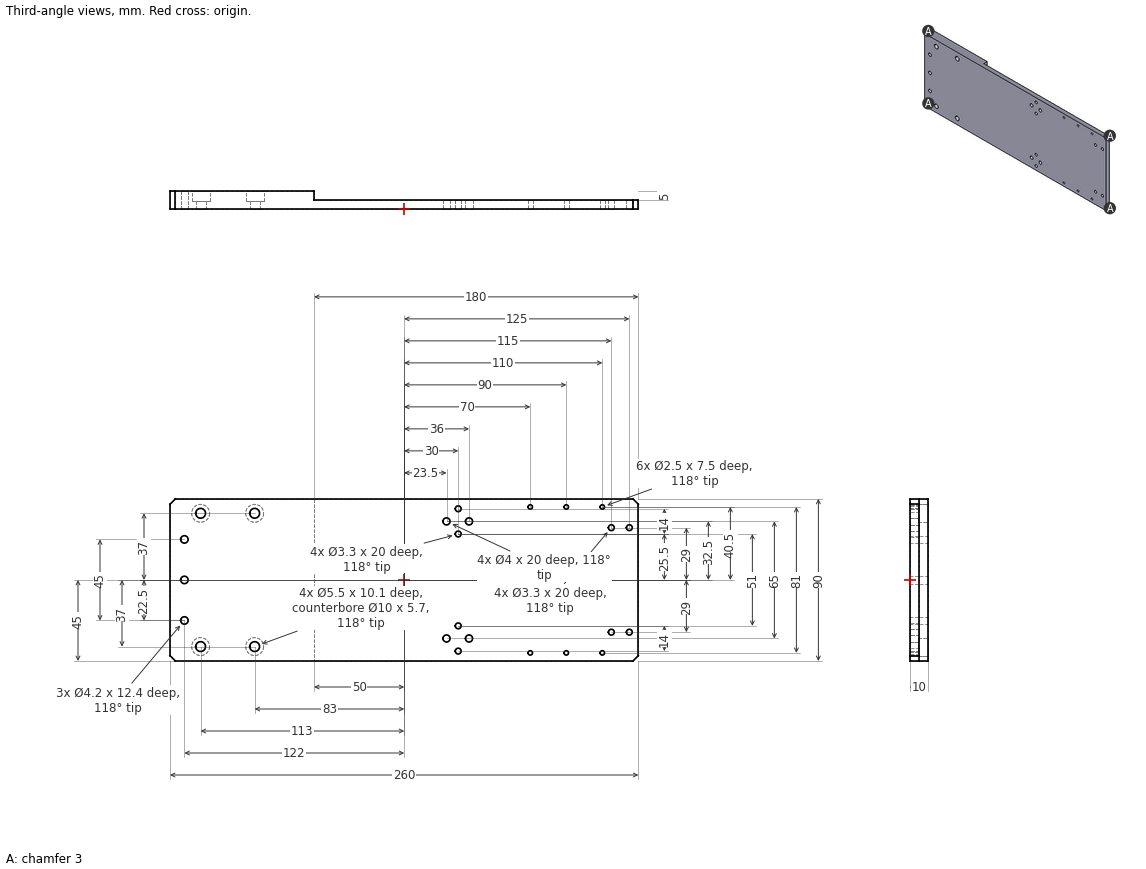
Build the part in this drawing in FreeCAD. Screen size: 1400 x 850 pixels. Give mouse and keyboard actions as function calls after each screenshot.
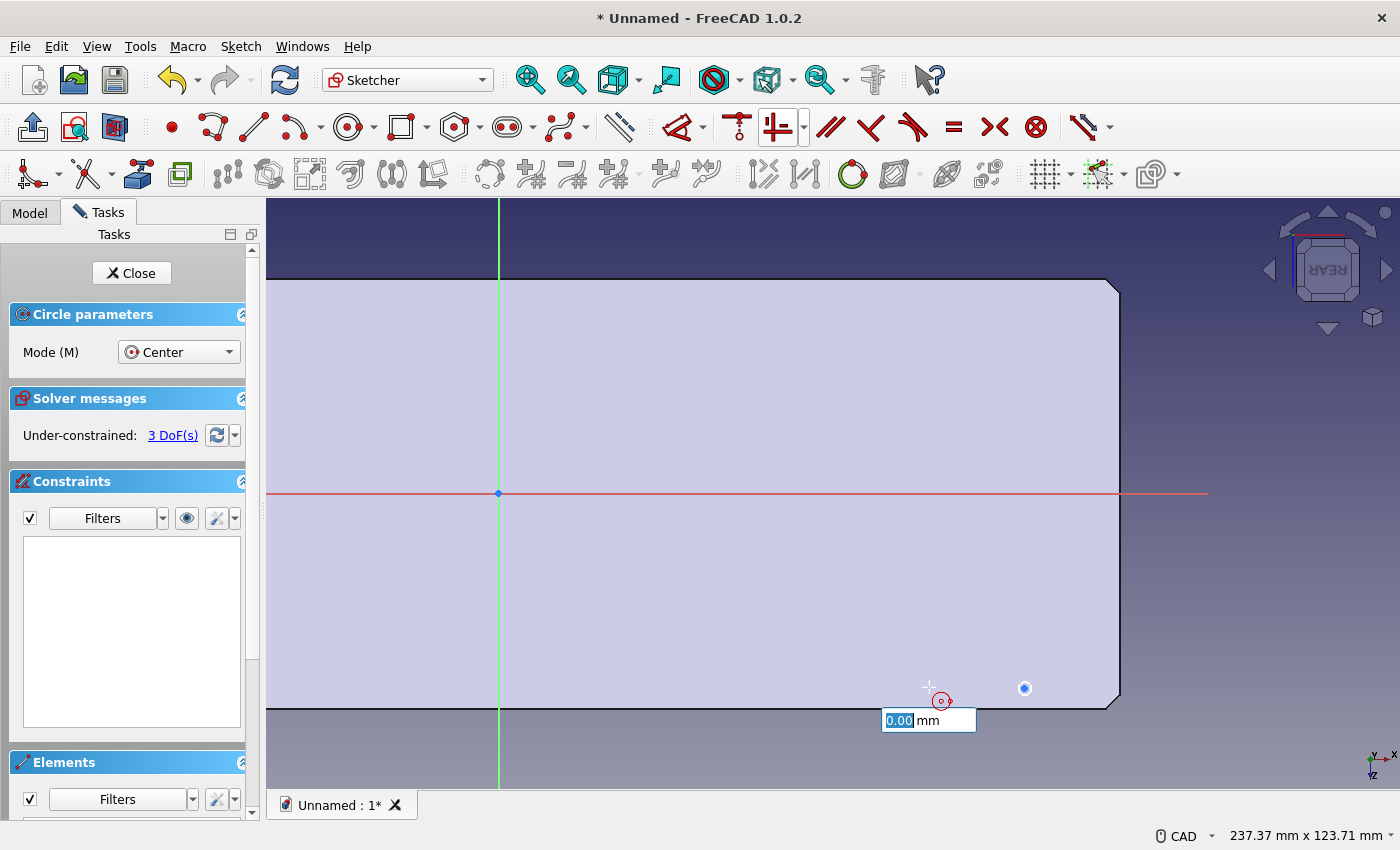
scroll(933, 683, up, 5)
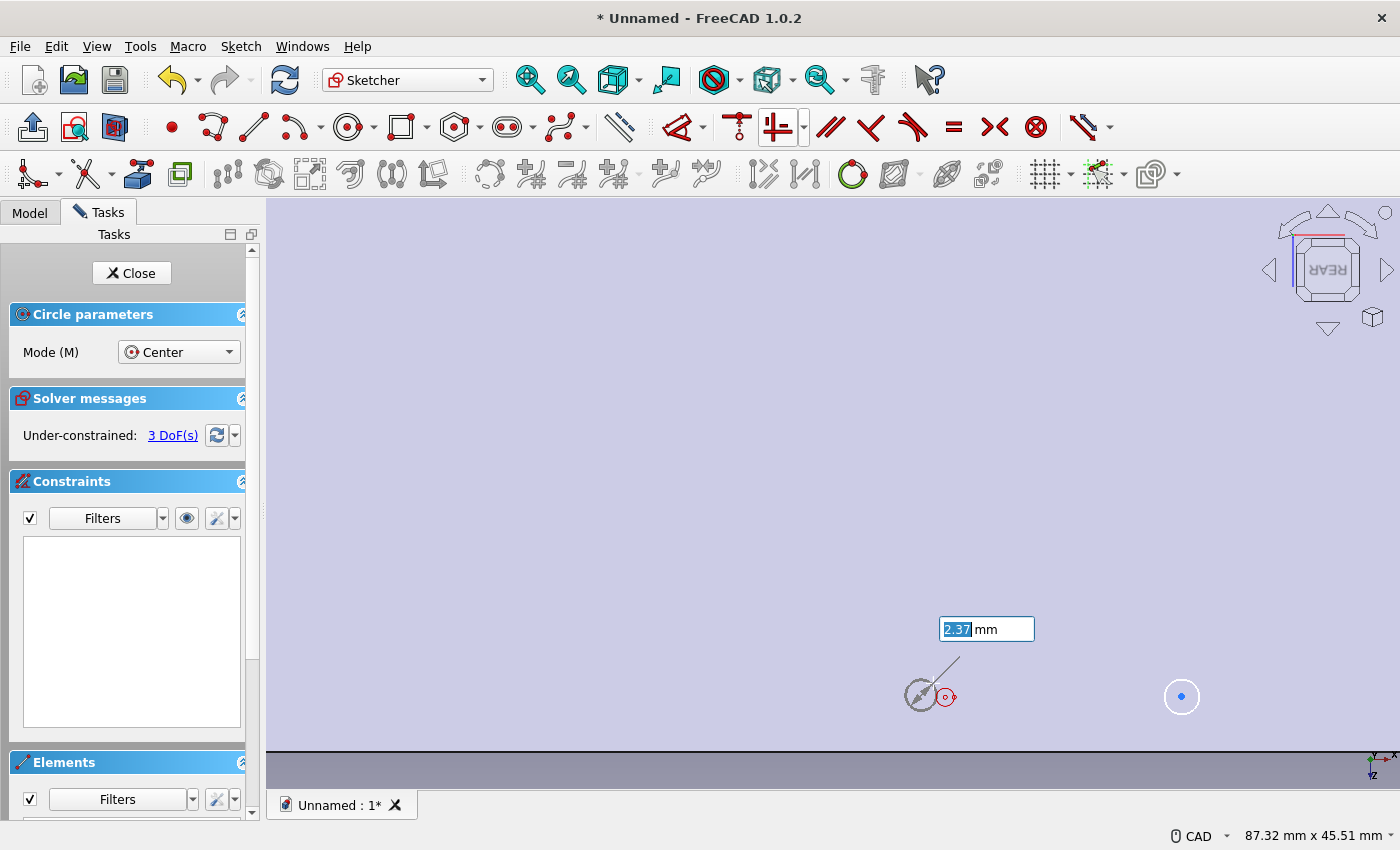
click(932, 682)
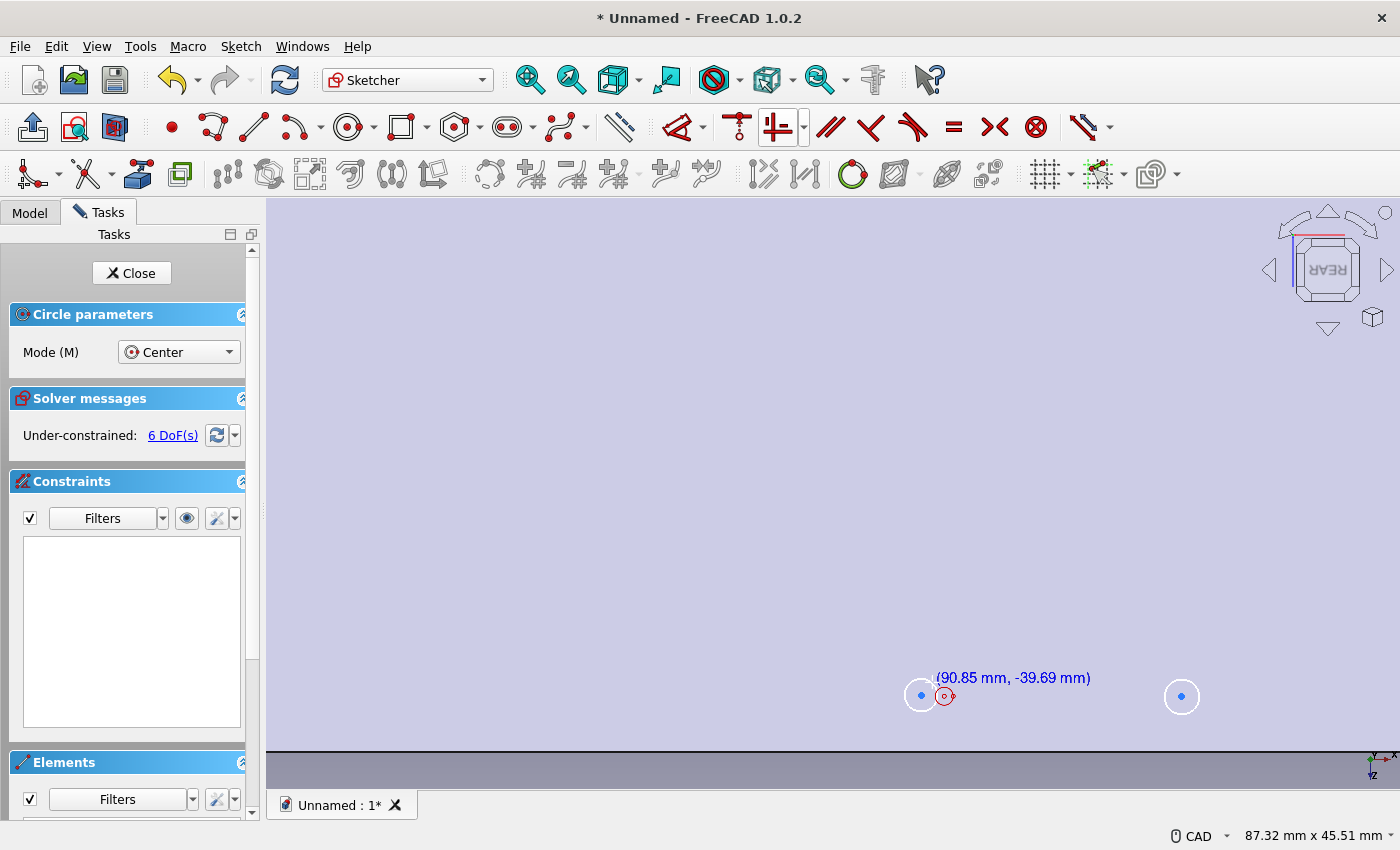
scroll(661, 694, up, 2)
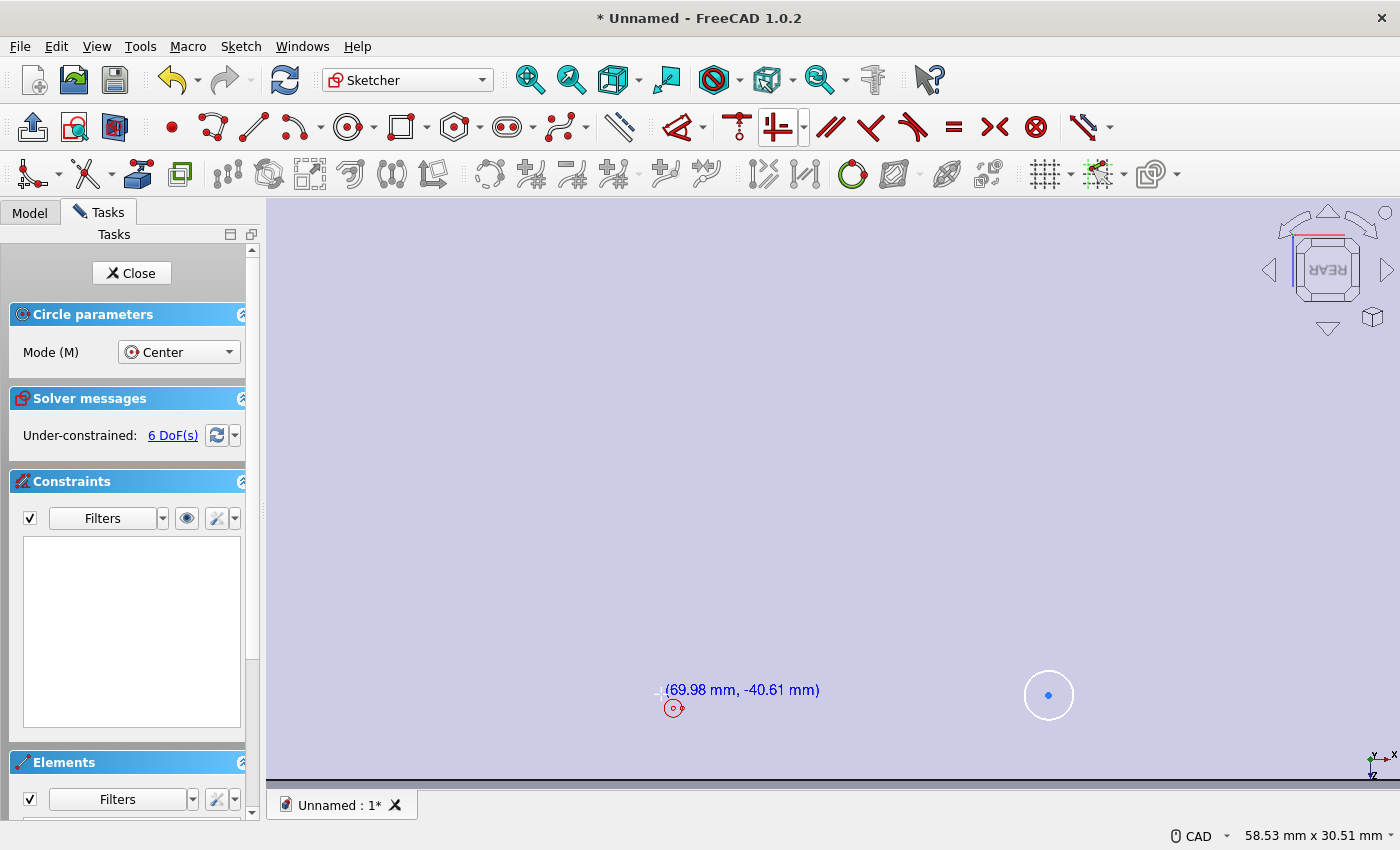
scroll(889, 685, down, 7)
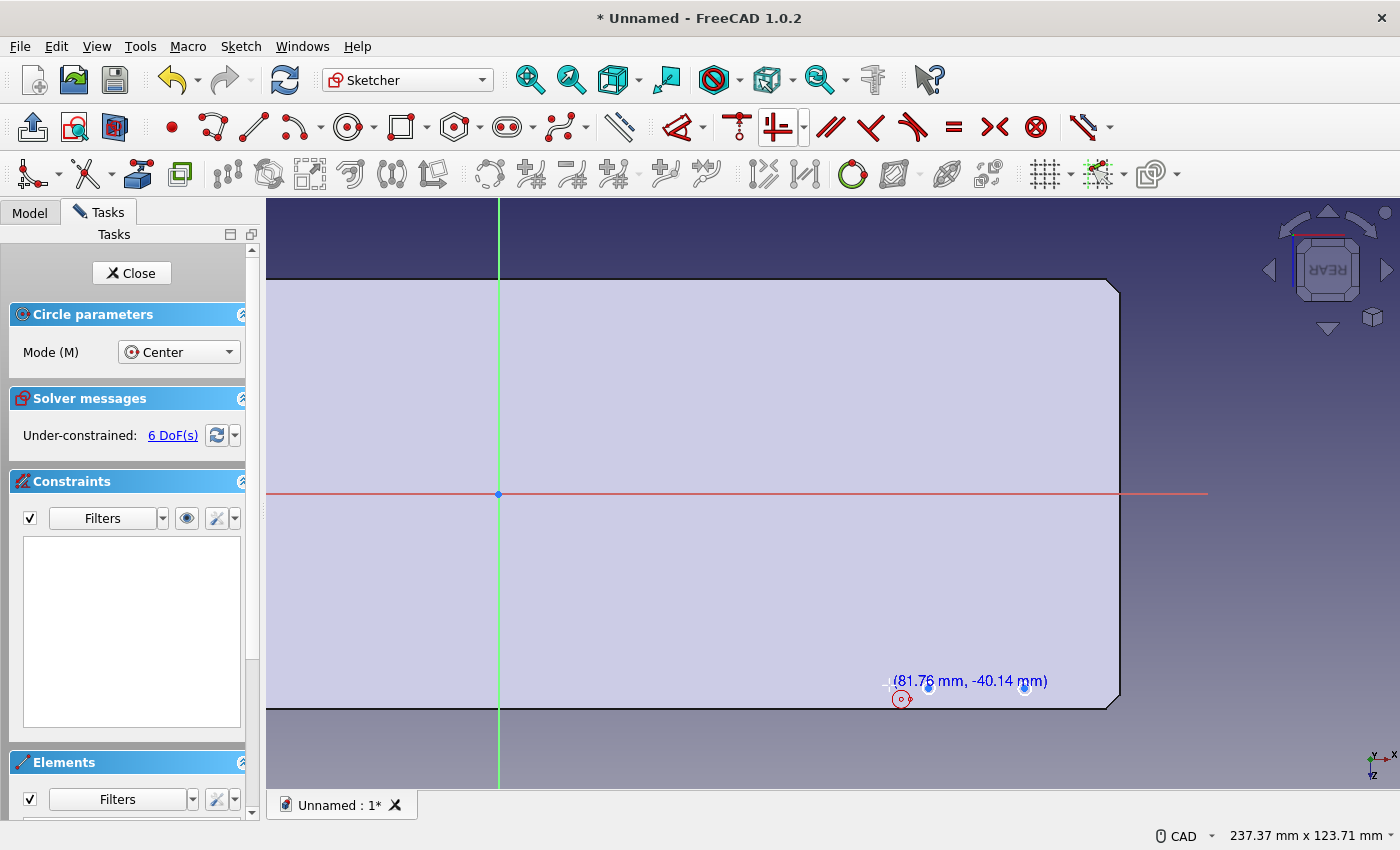
click(833, 688)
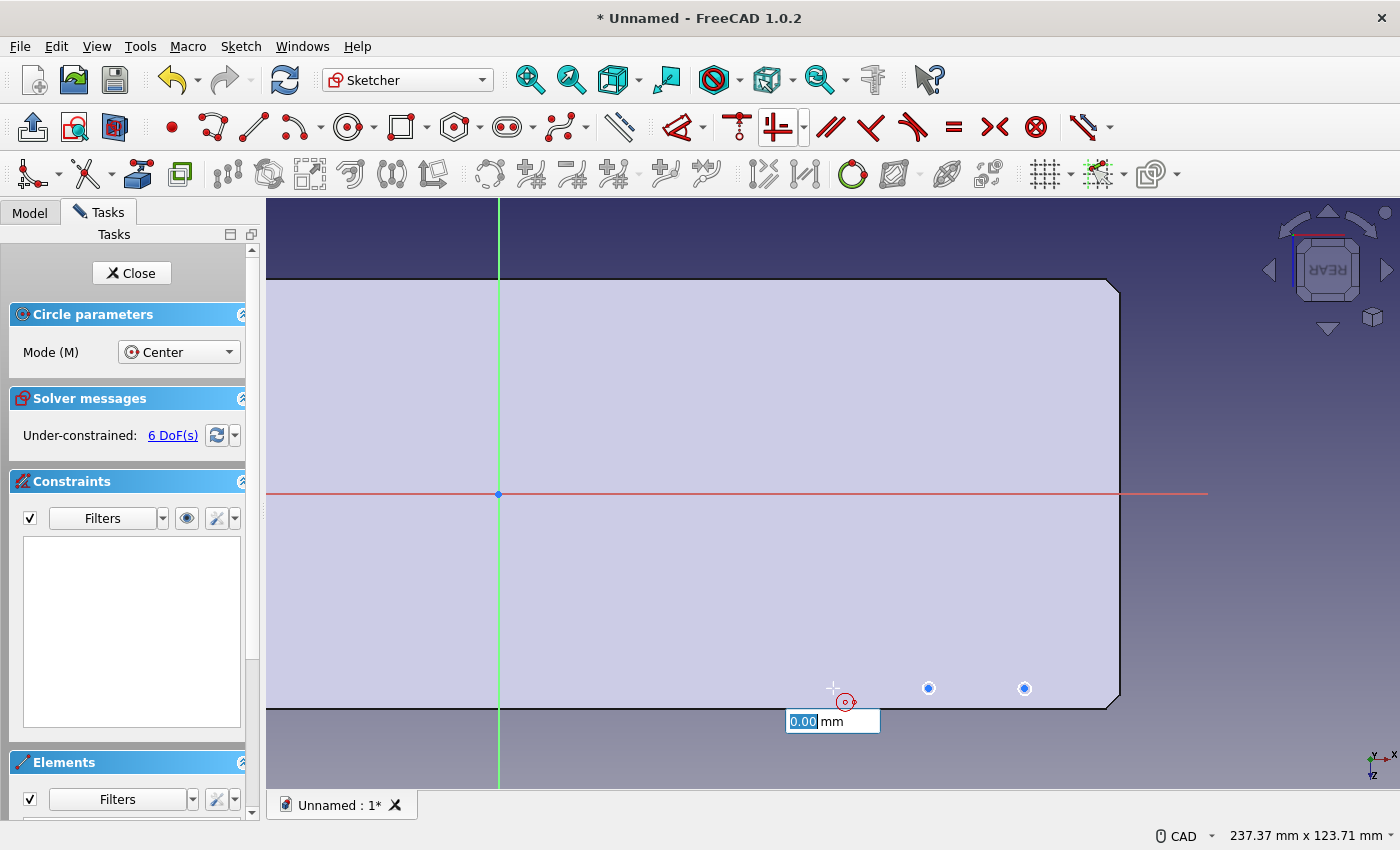
scroll(837, 683, up, 5)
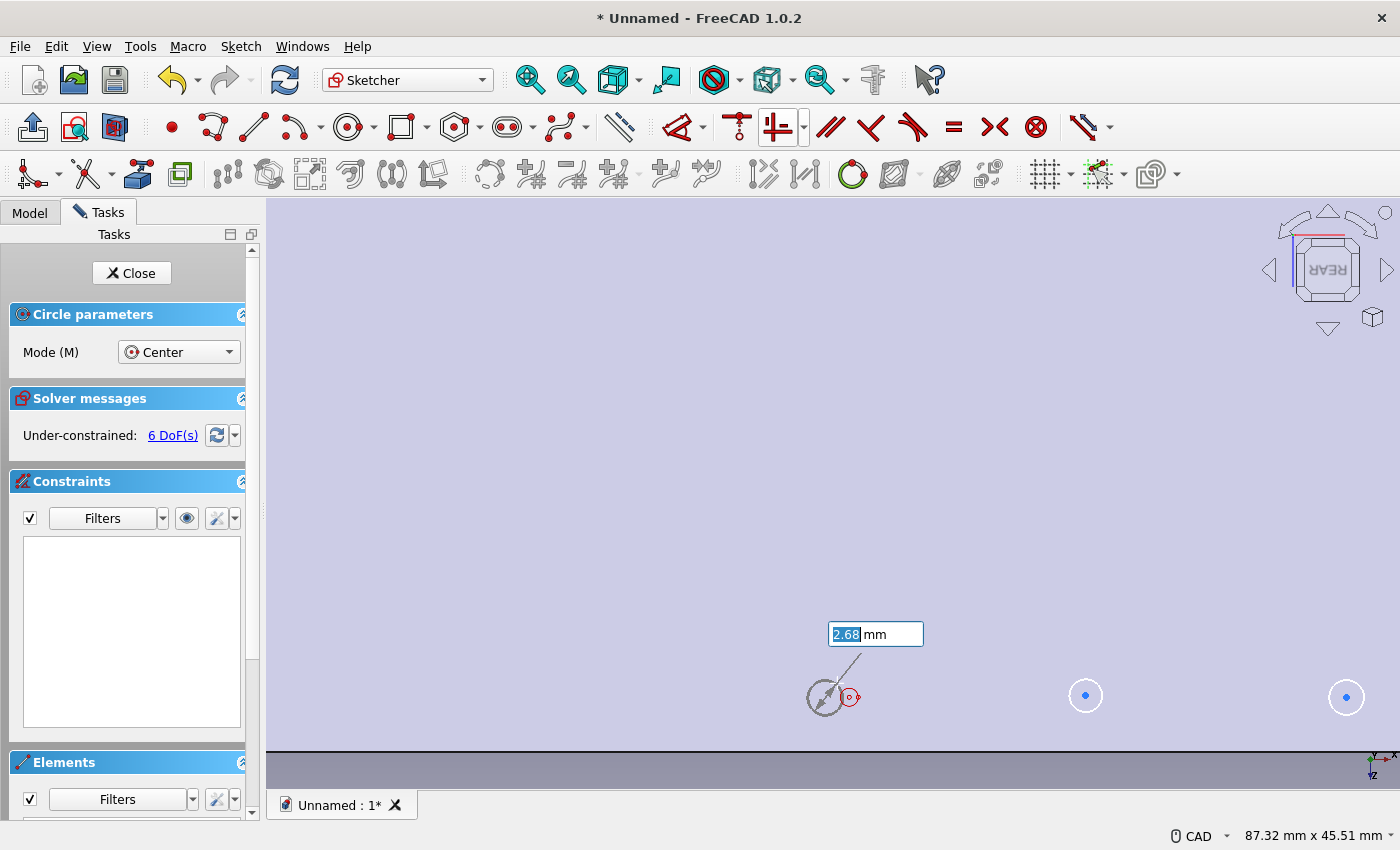
click(837, 683)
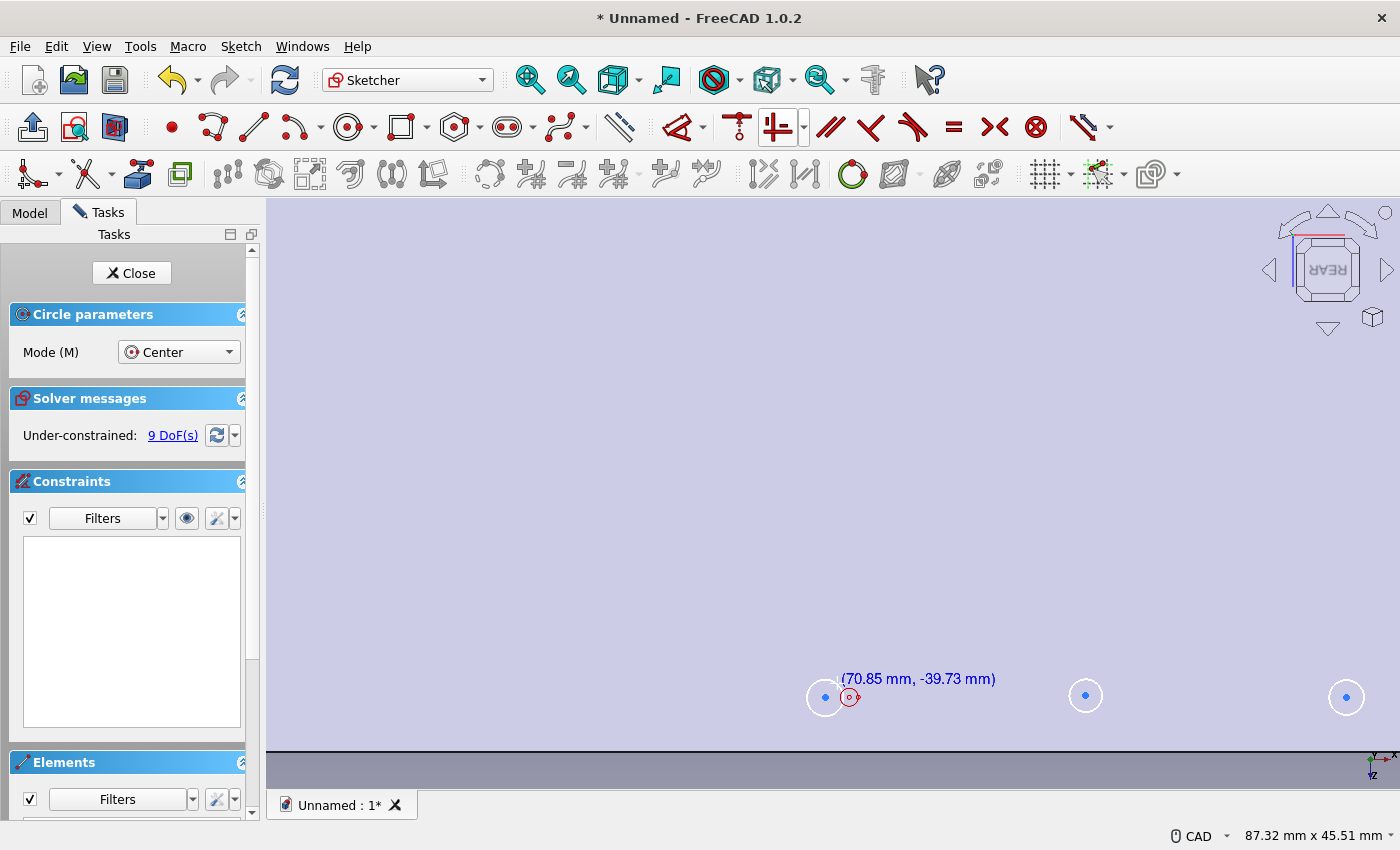
scroll(837, 683, down, 5)